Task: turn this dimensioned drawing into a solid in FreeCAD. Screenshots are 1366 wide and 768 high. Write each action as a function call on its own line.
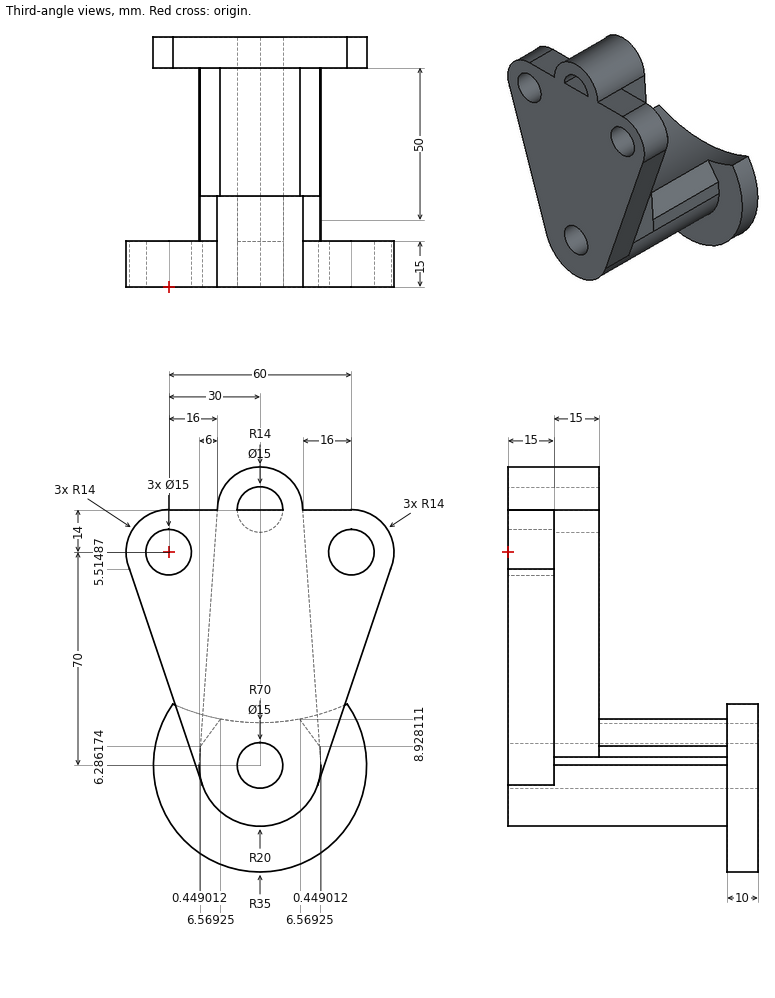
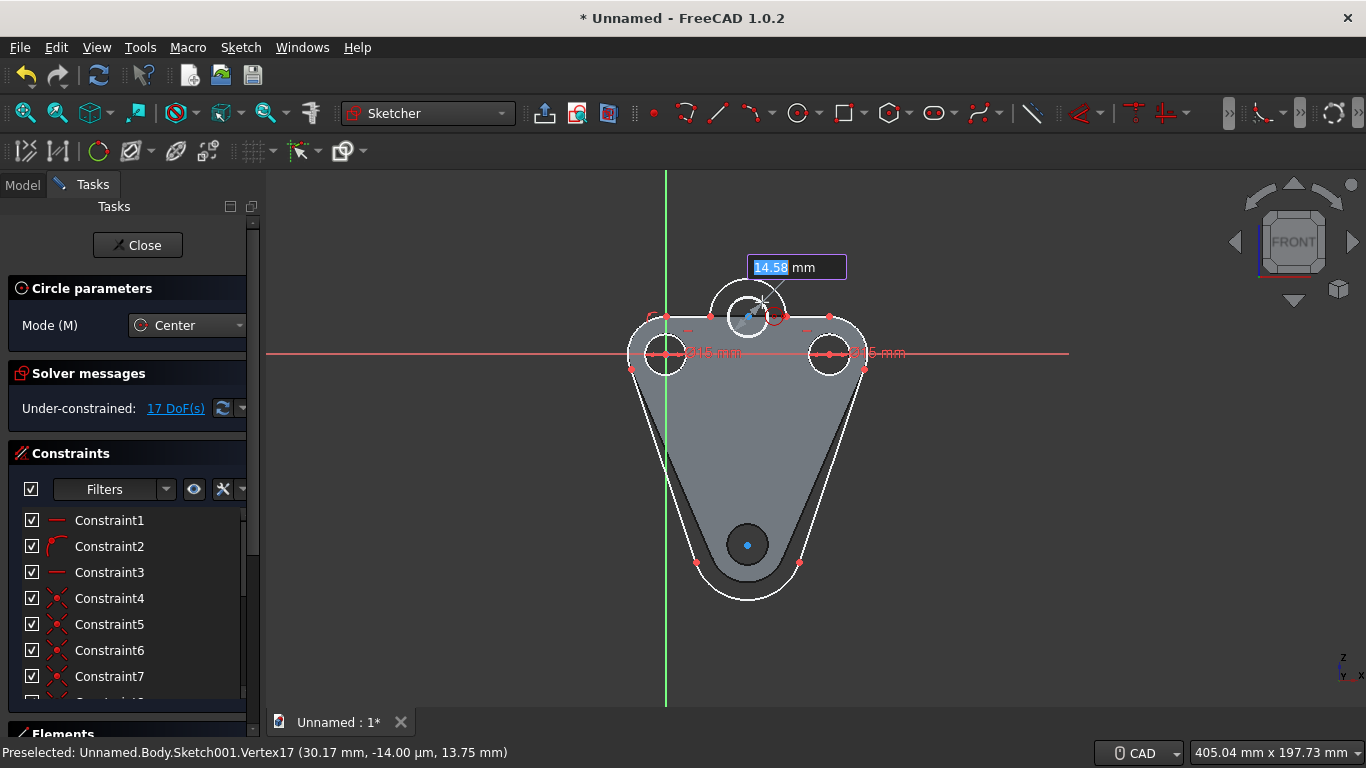
text(15)
key(Return)
key(Escape)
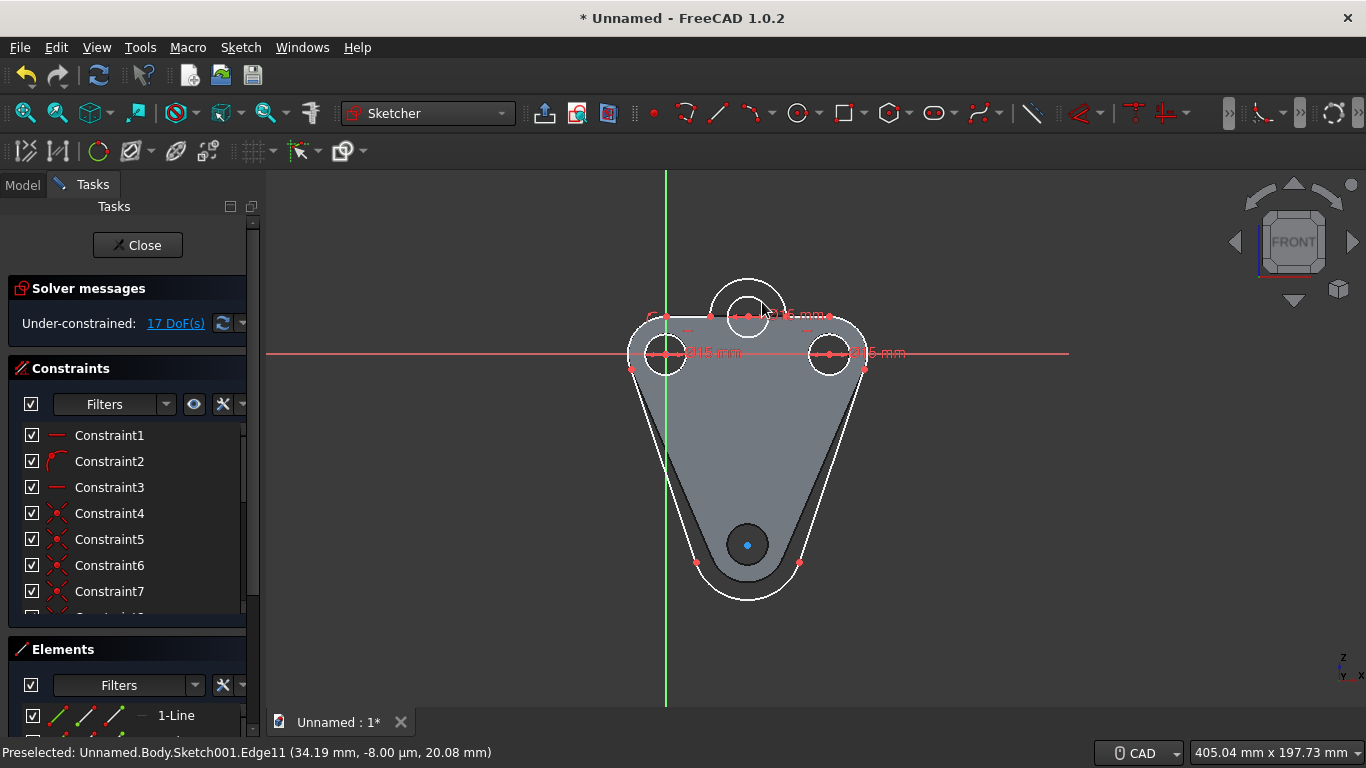
click(651, 428)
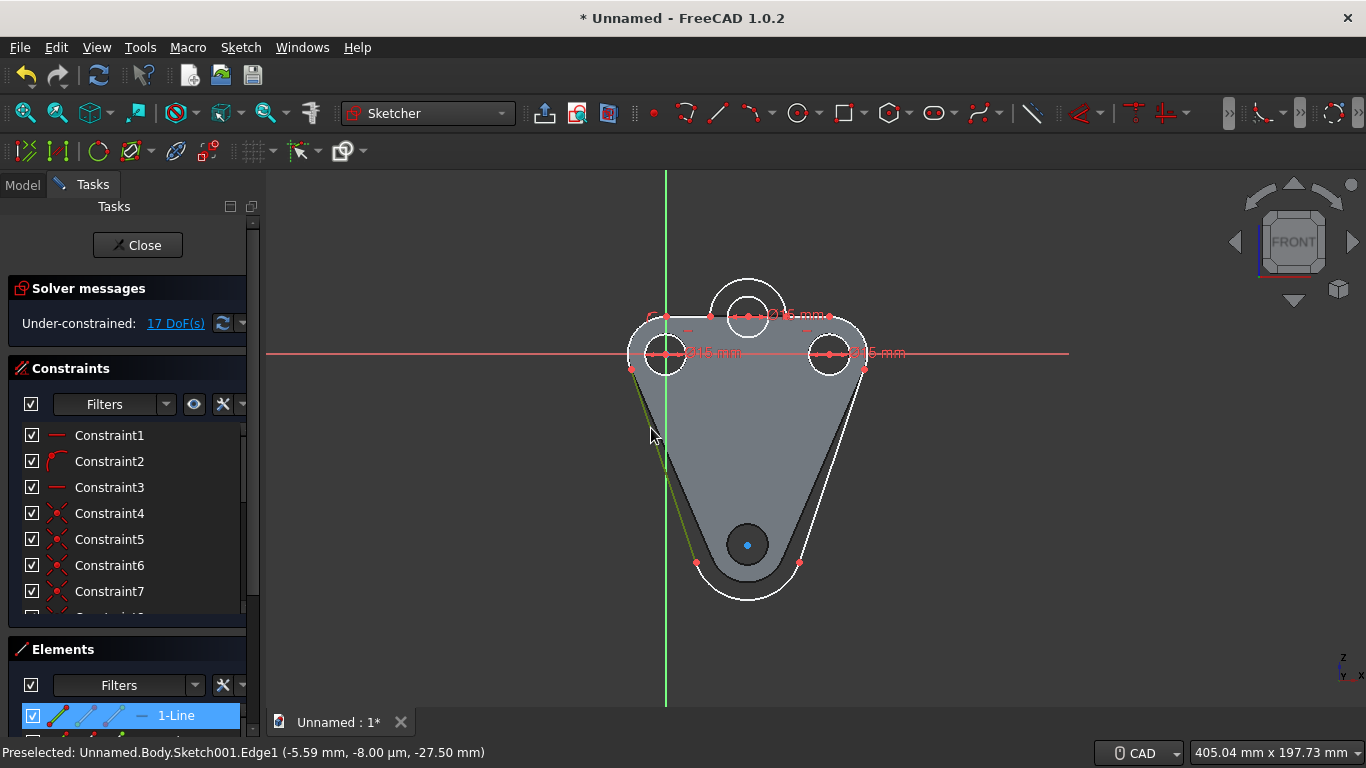
click(722, 593)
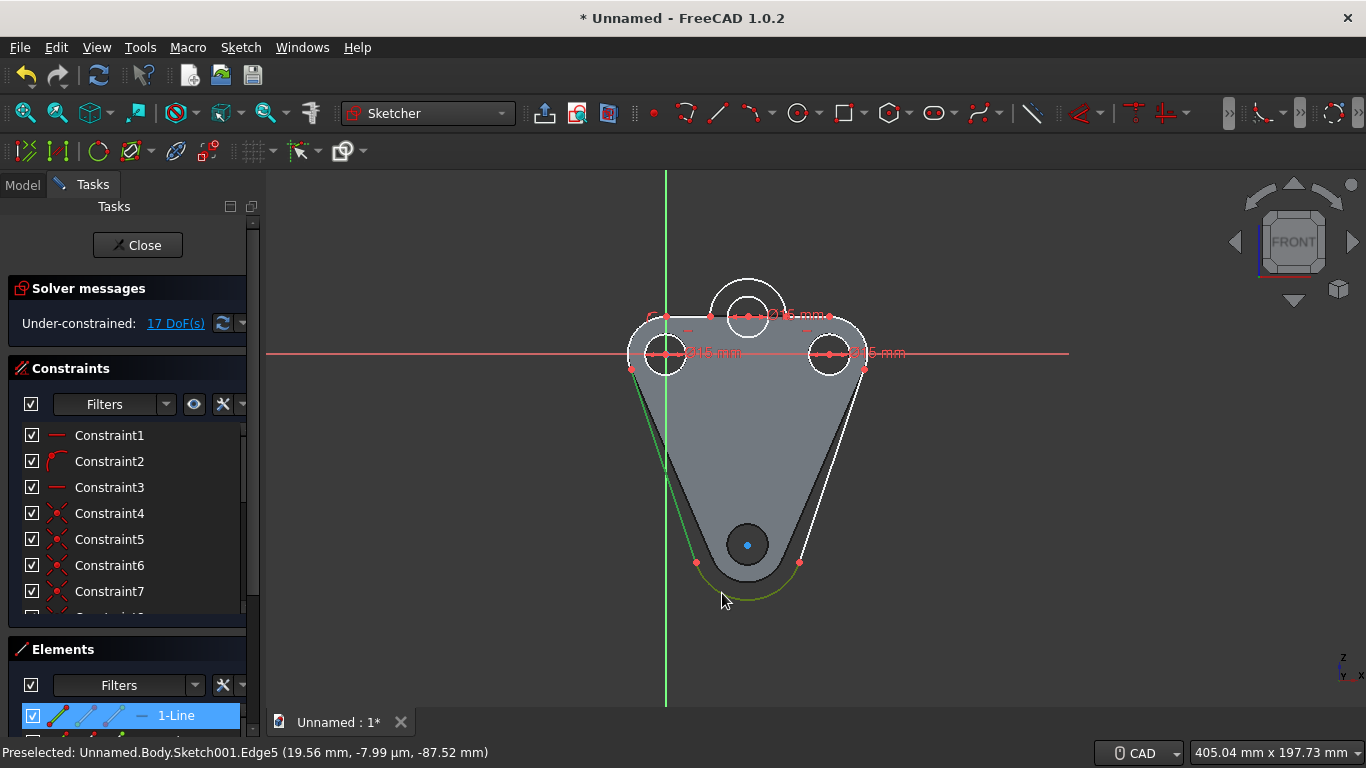
key(t)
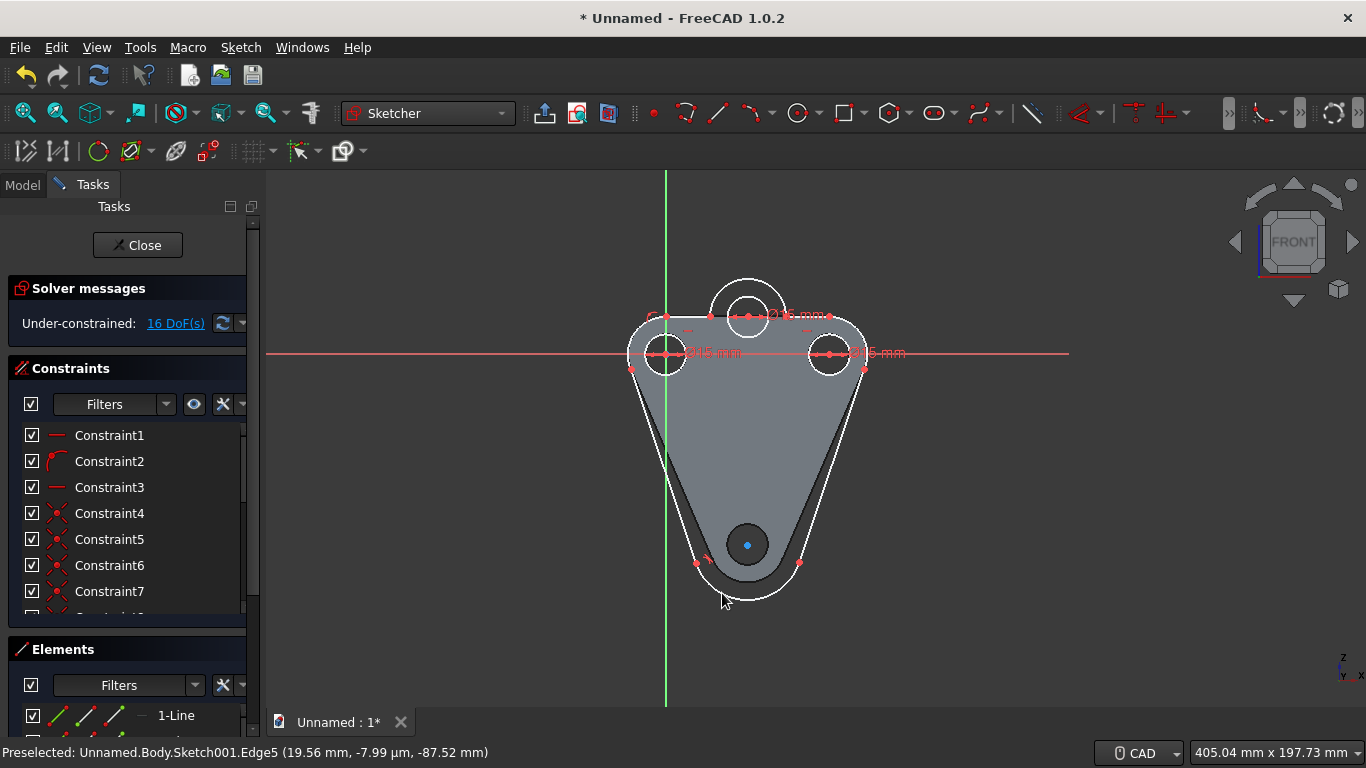
click(819, 505)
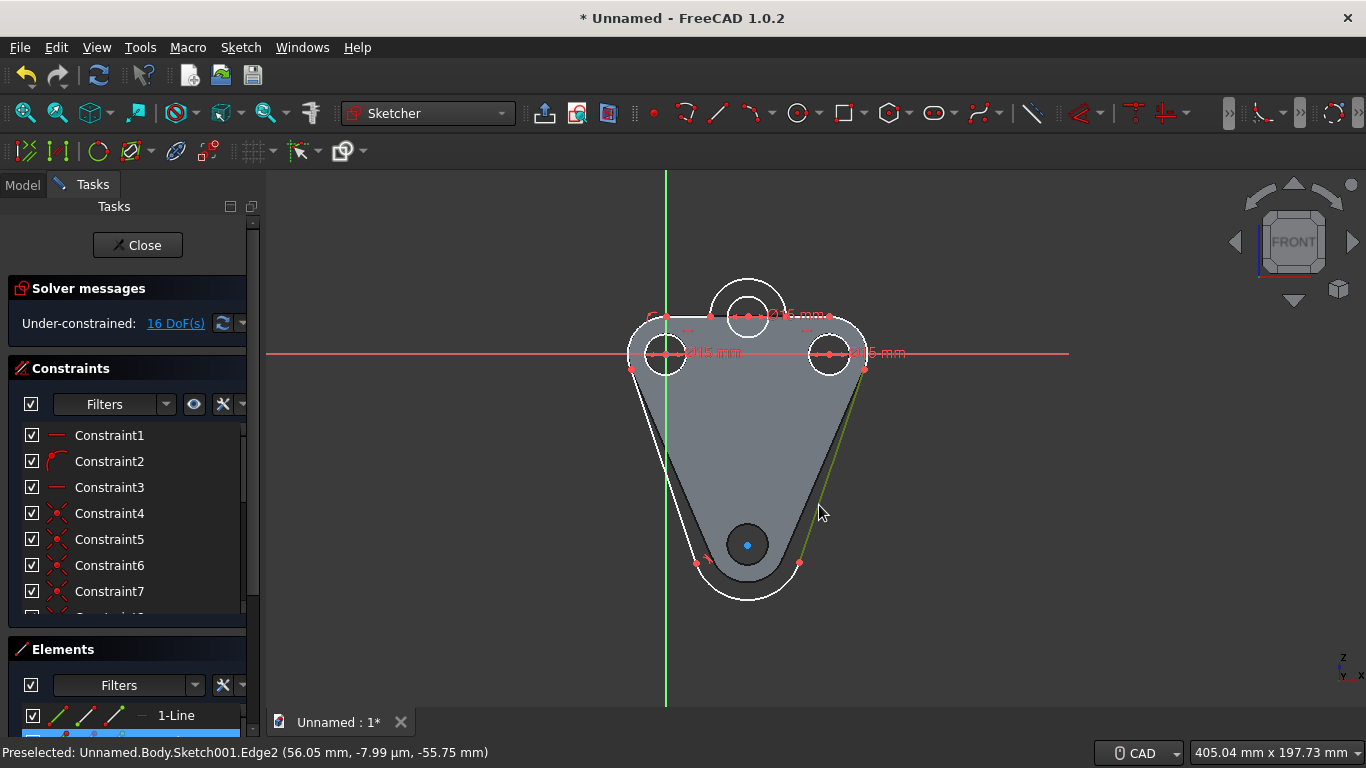
click(722, 593)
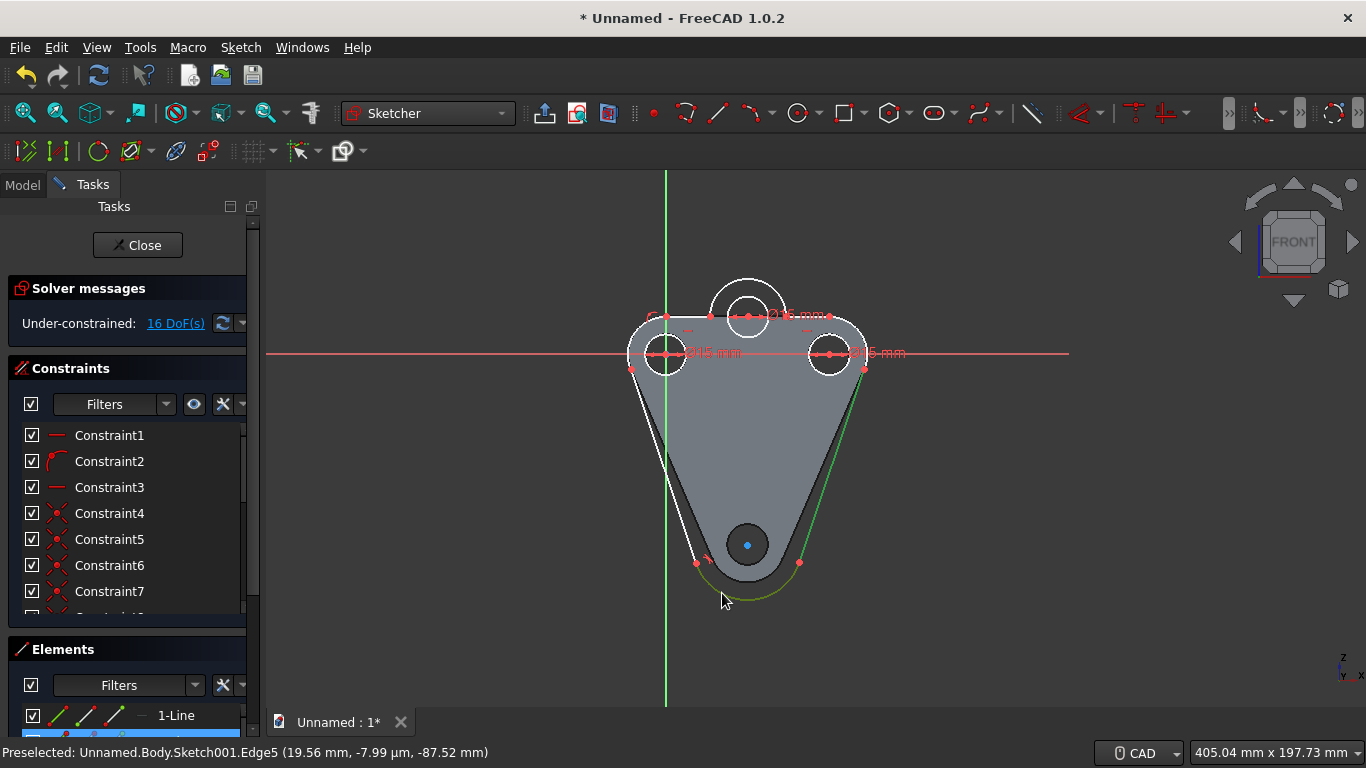
key(t)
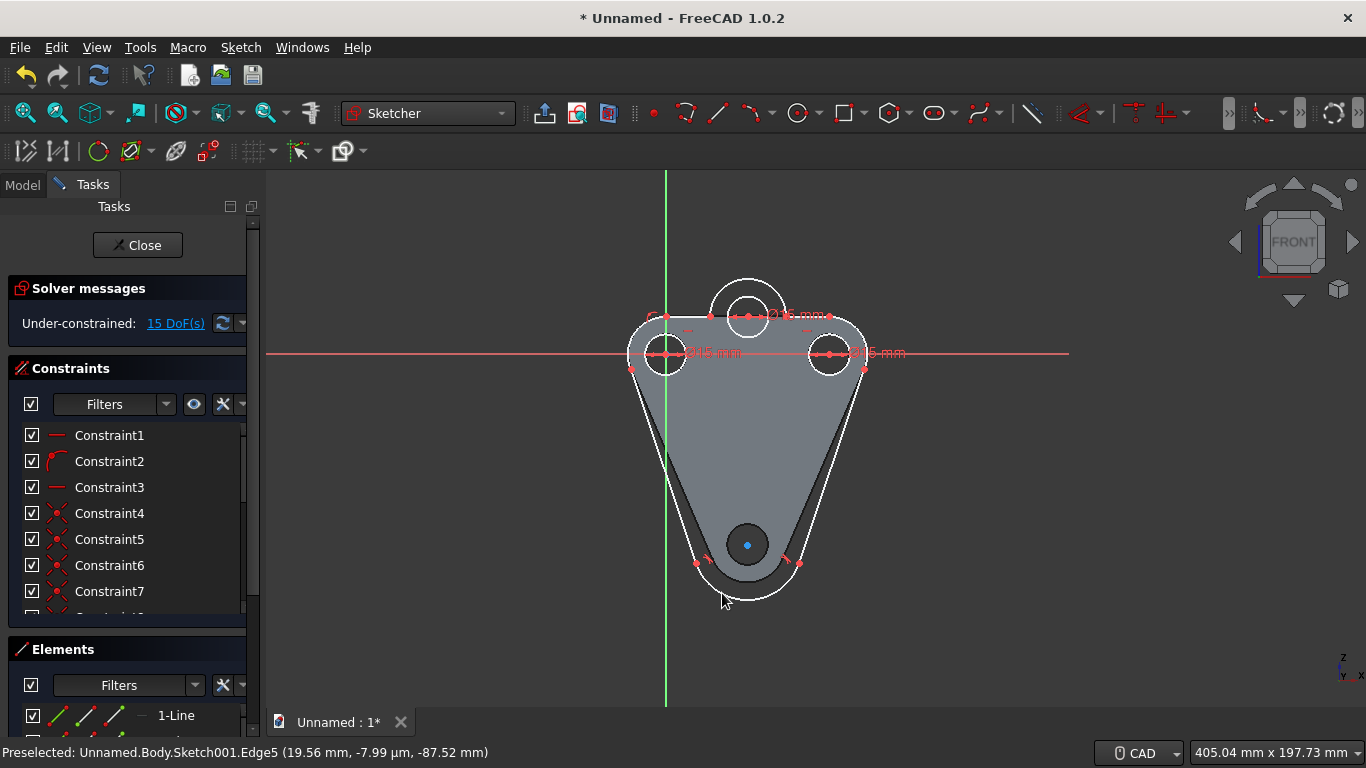
scroll(816, 317, up, 4)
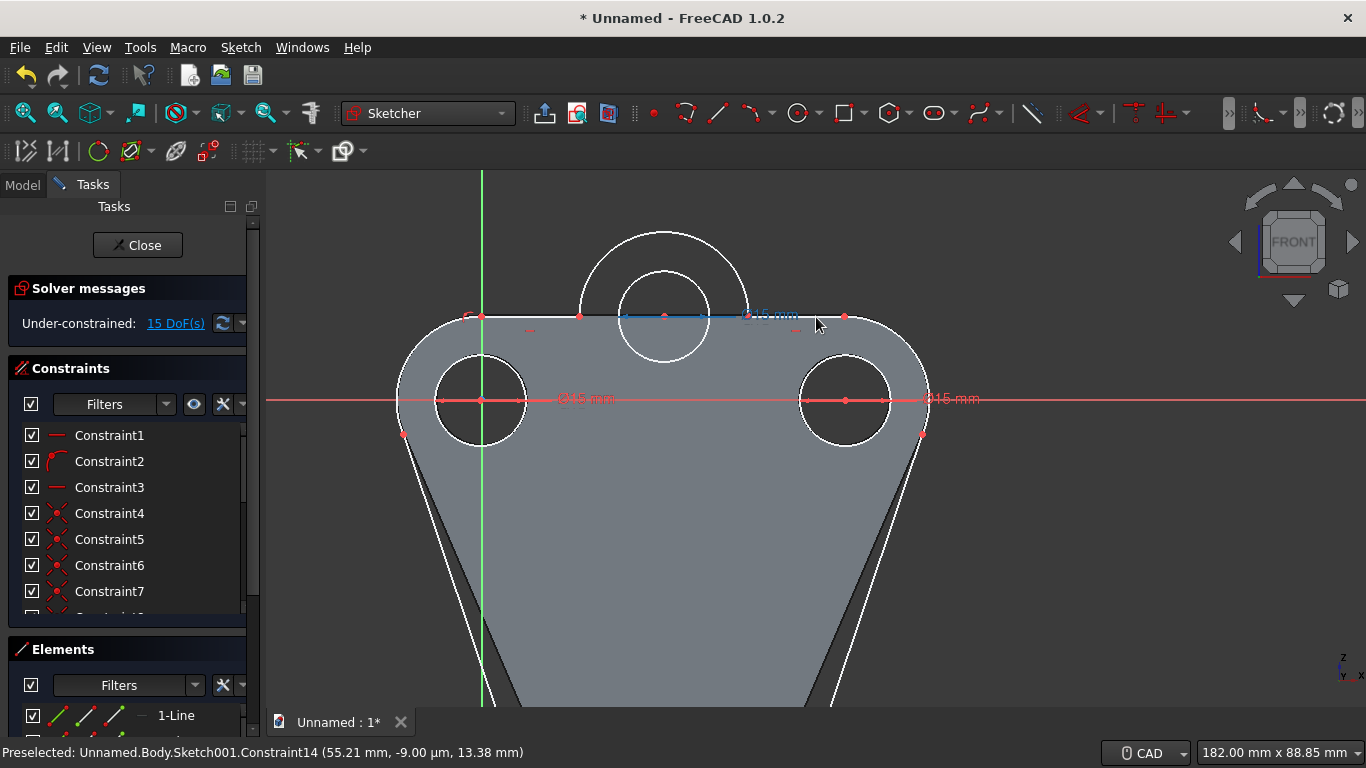
click(816, 317)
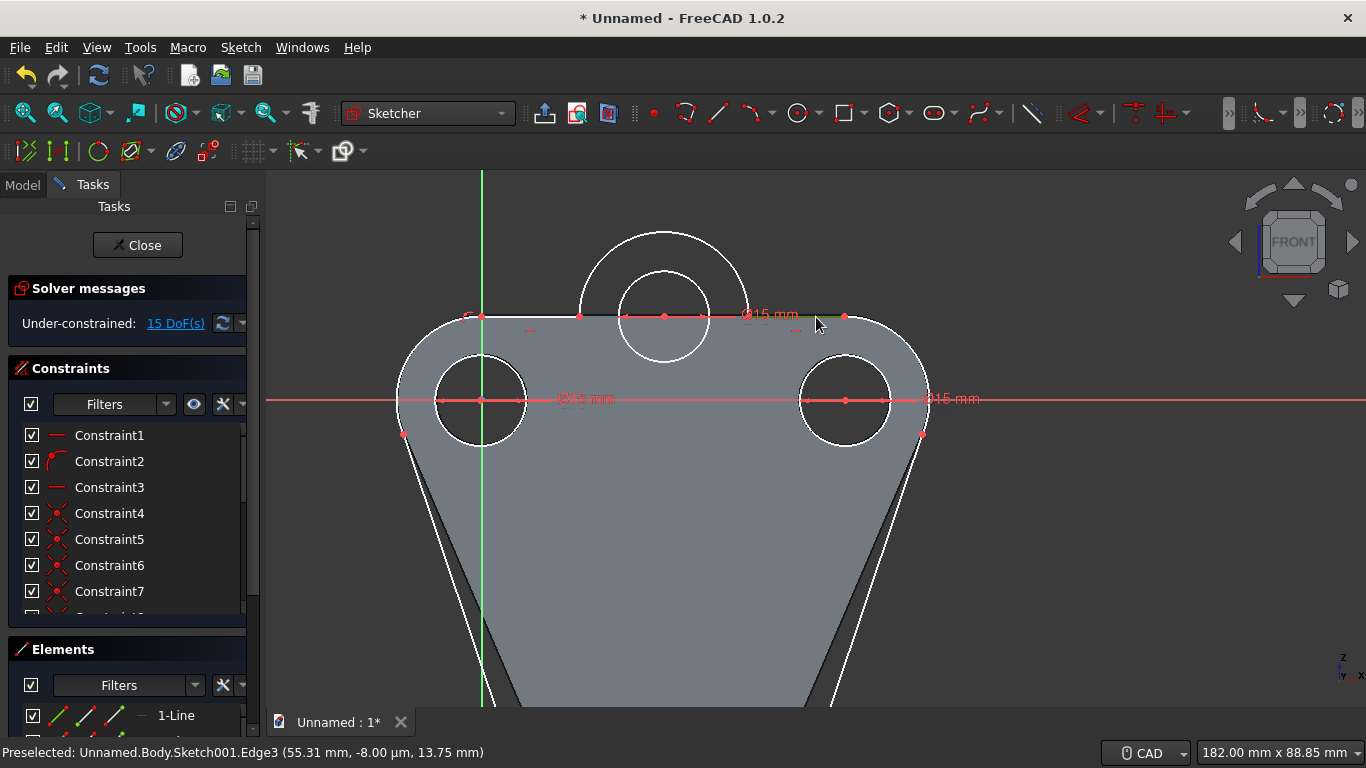
click(928, 385)